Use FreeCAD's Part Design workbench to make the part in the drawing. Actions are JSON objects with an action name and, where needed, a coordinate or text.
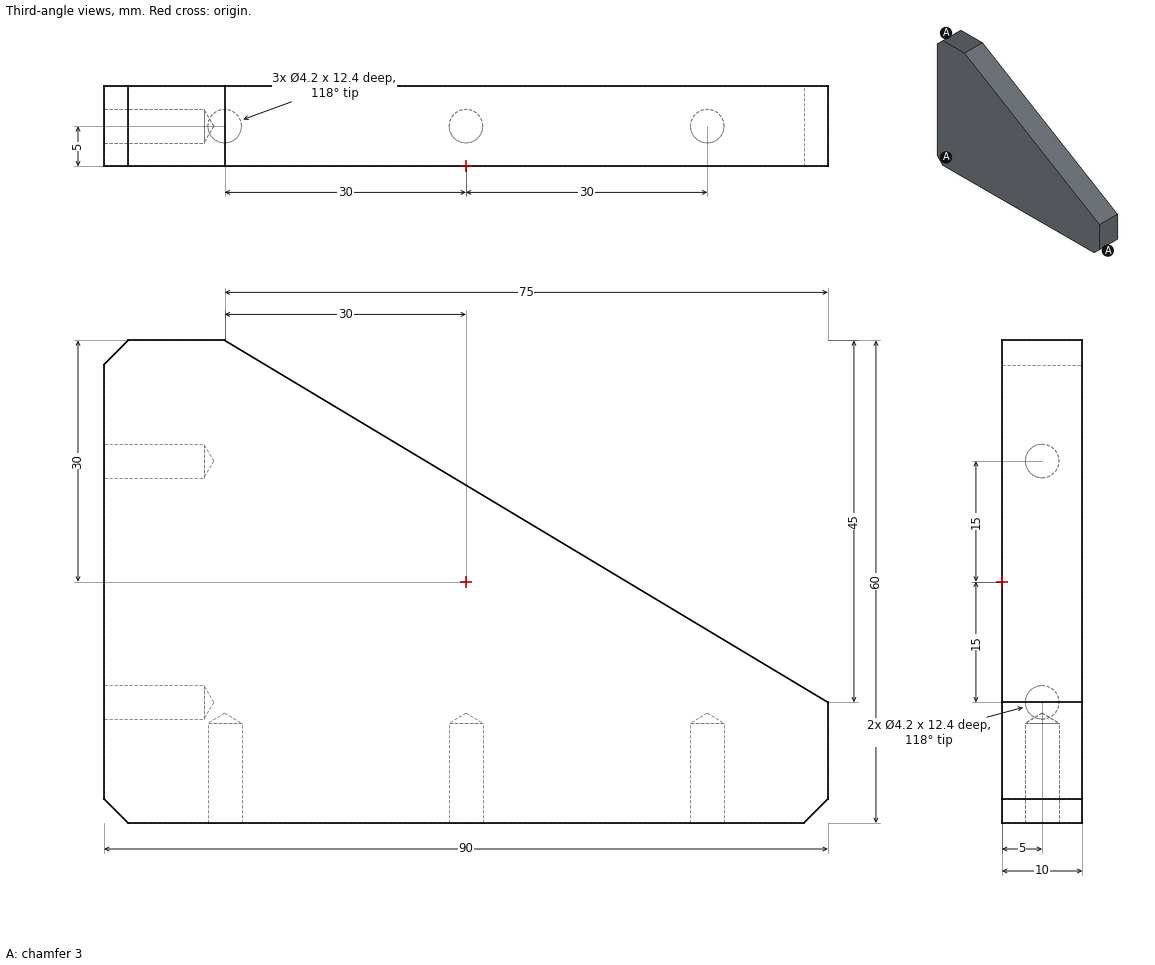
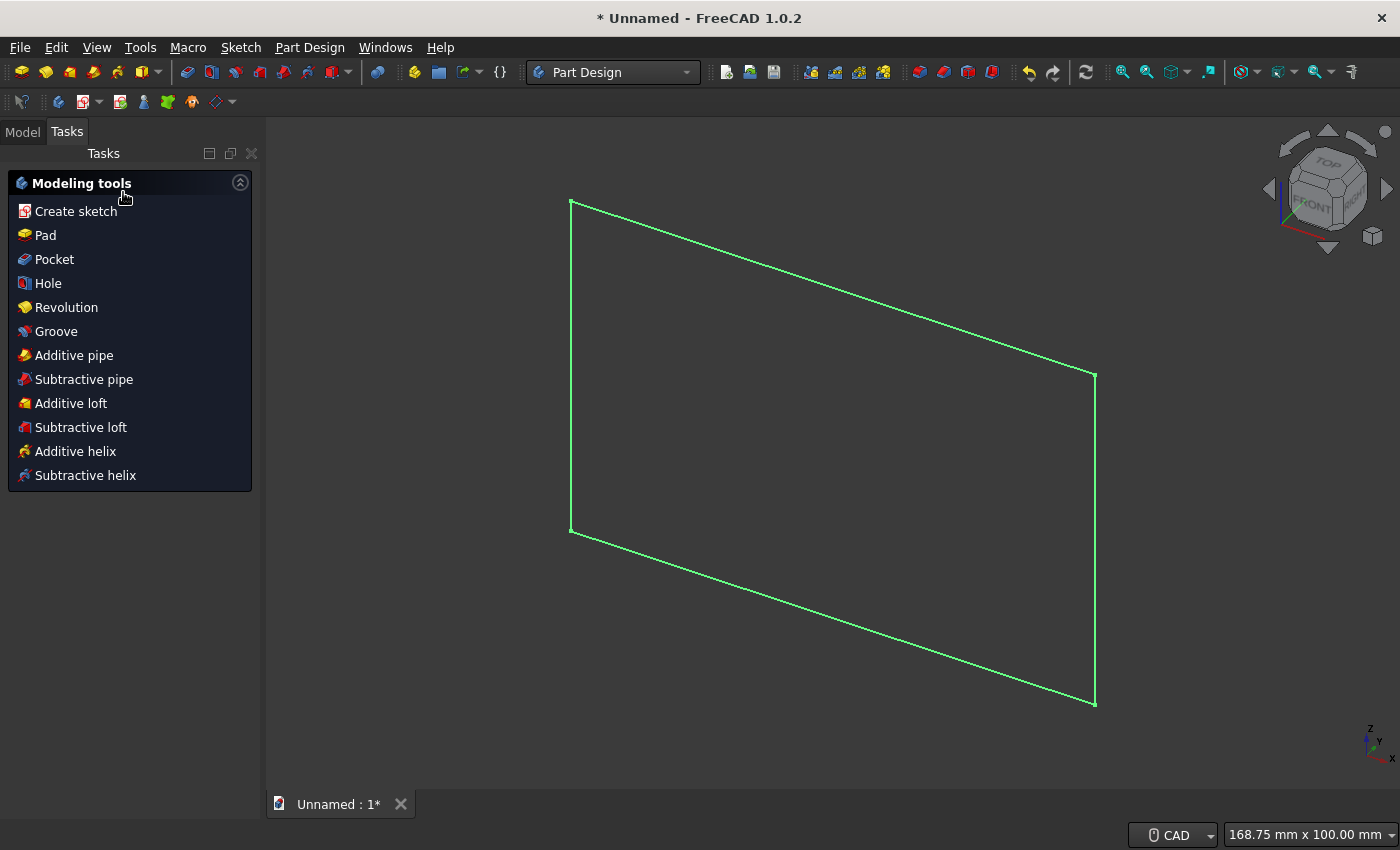
{"action": "left_click", "coordinate": [22, 72]}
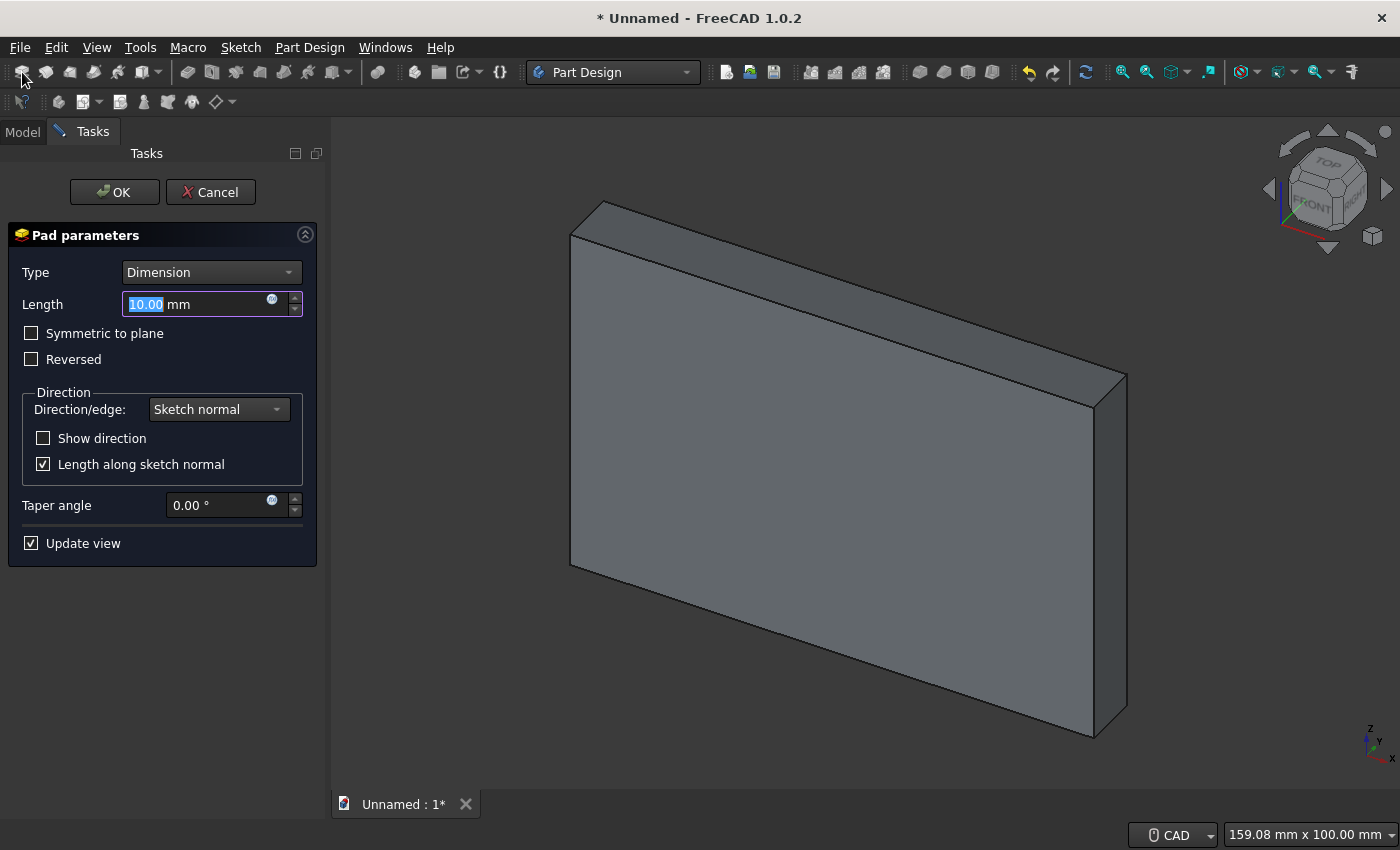
{"action": "type", "text": "10"}
{"action": "key", "text": "Tab"}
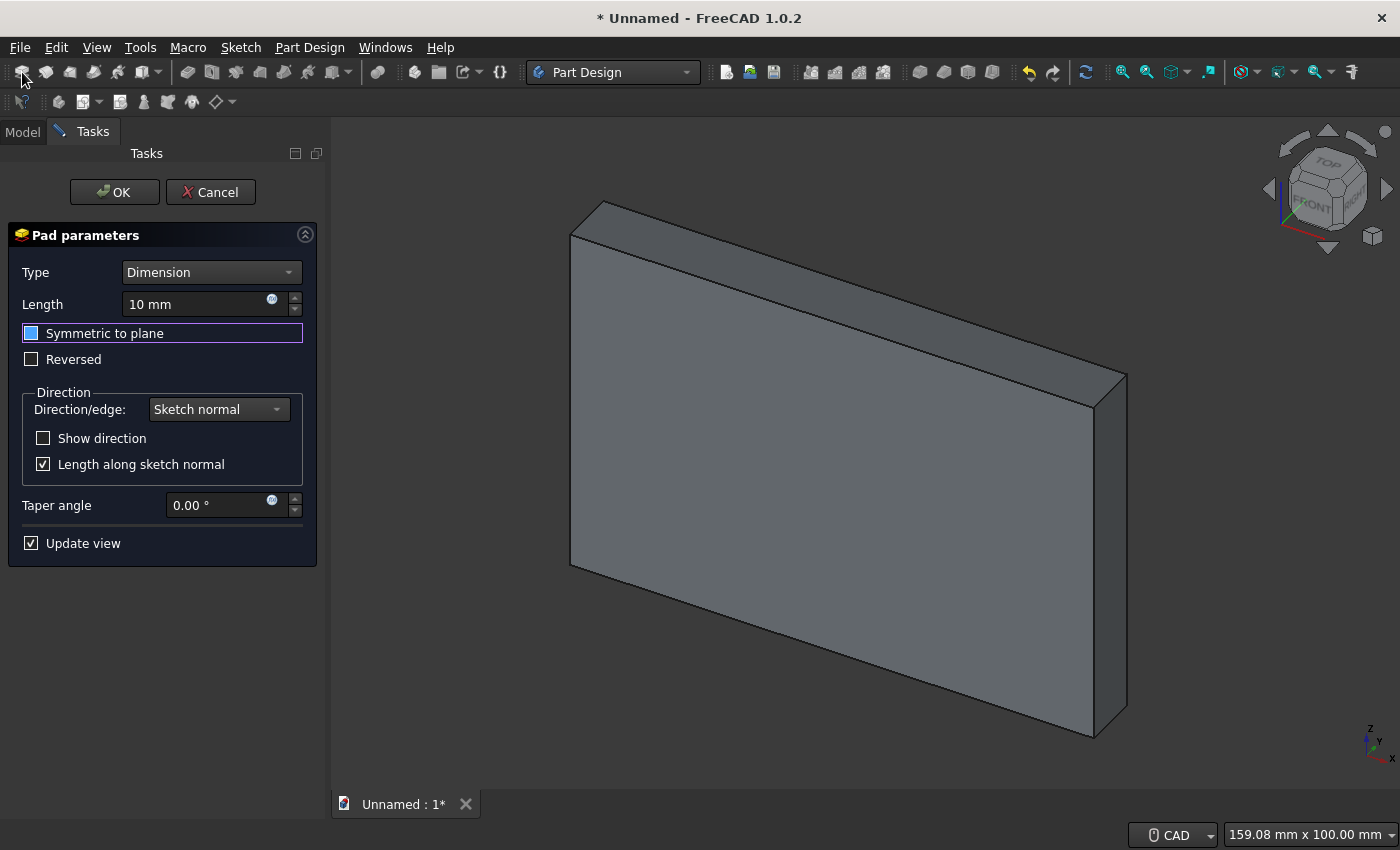
{"action": "left_click", "coordinate": [30, 359]}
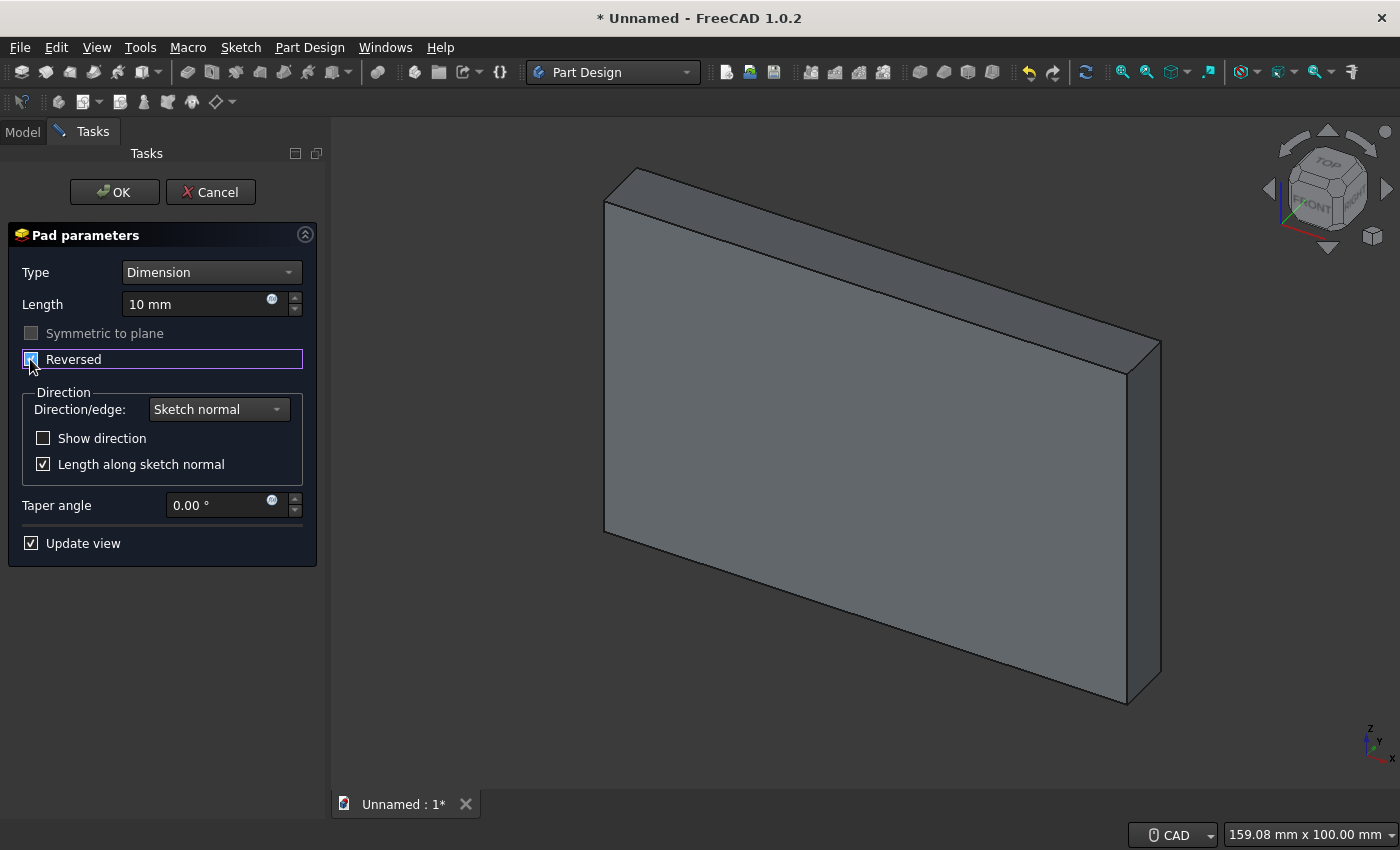
{"action": "left_click", "coordinate": [115, 192]}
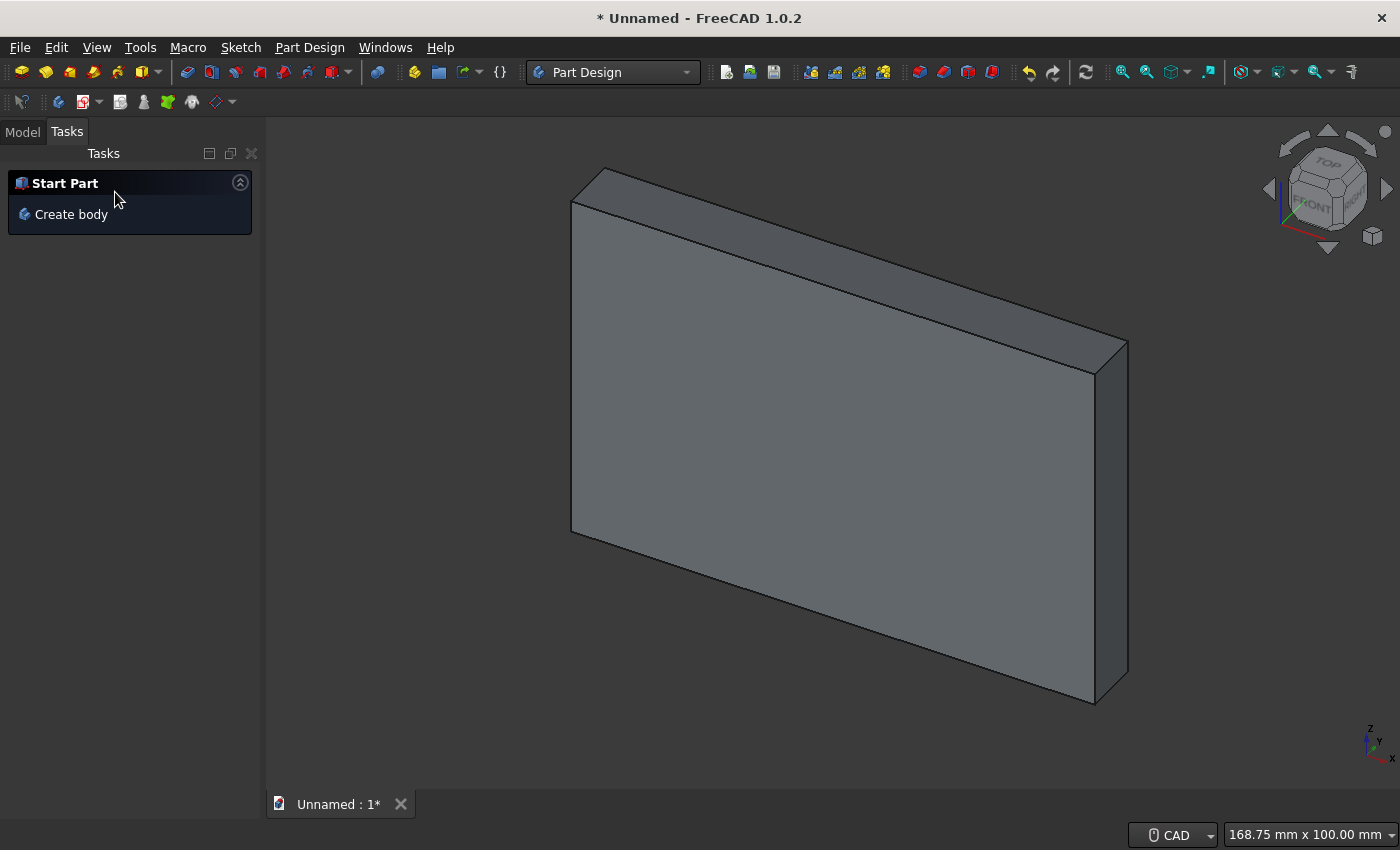
{"action": "key", "text": "4"}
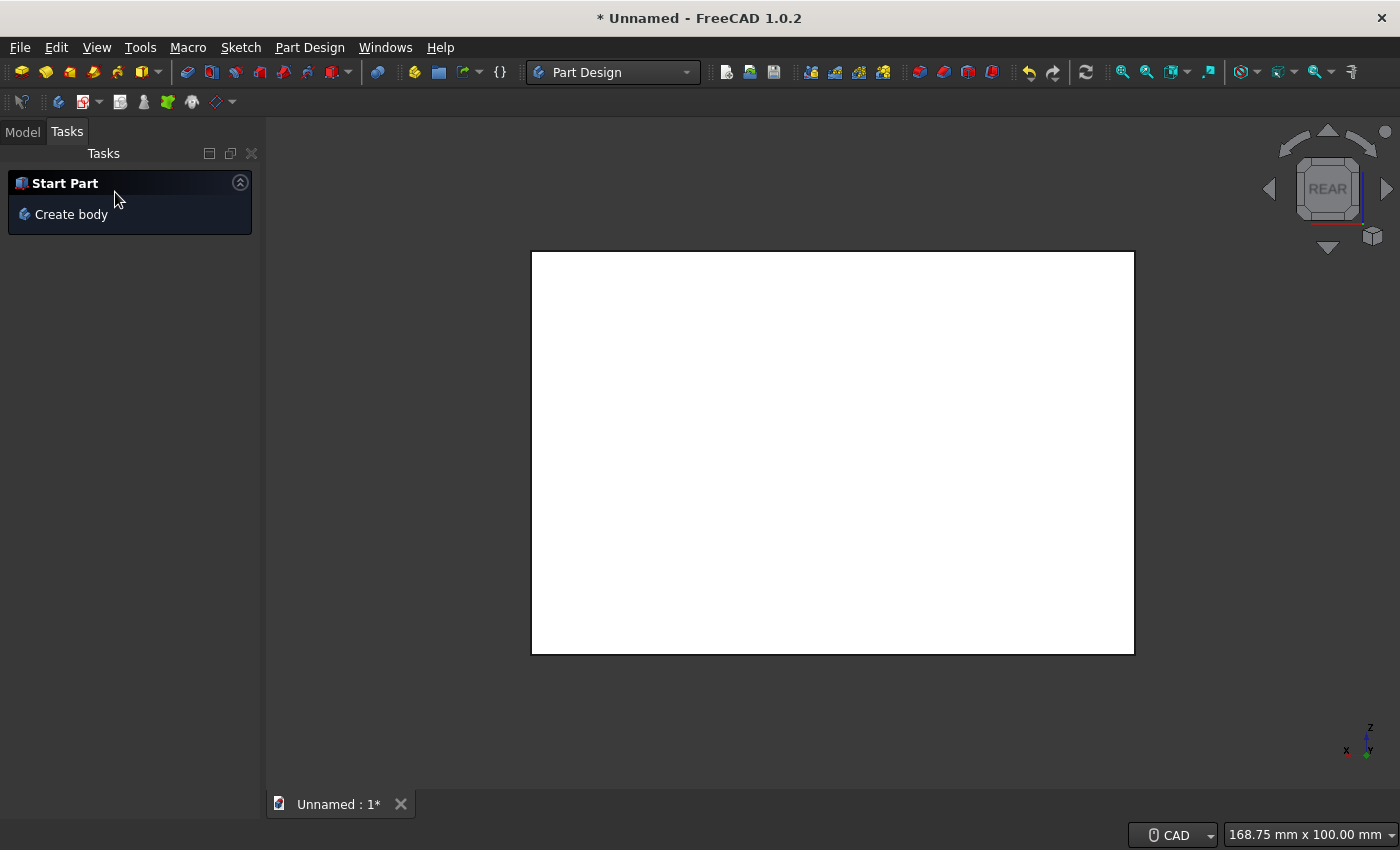
{"action": "left_click", "coordinate": [747, 452]}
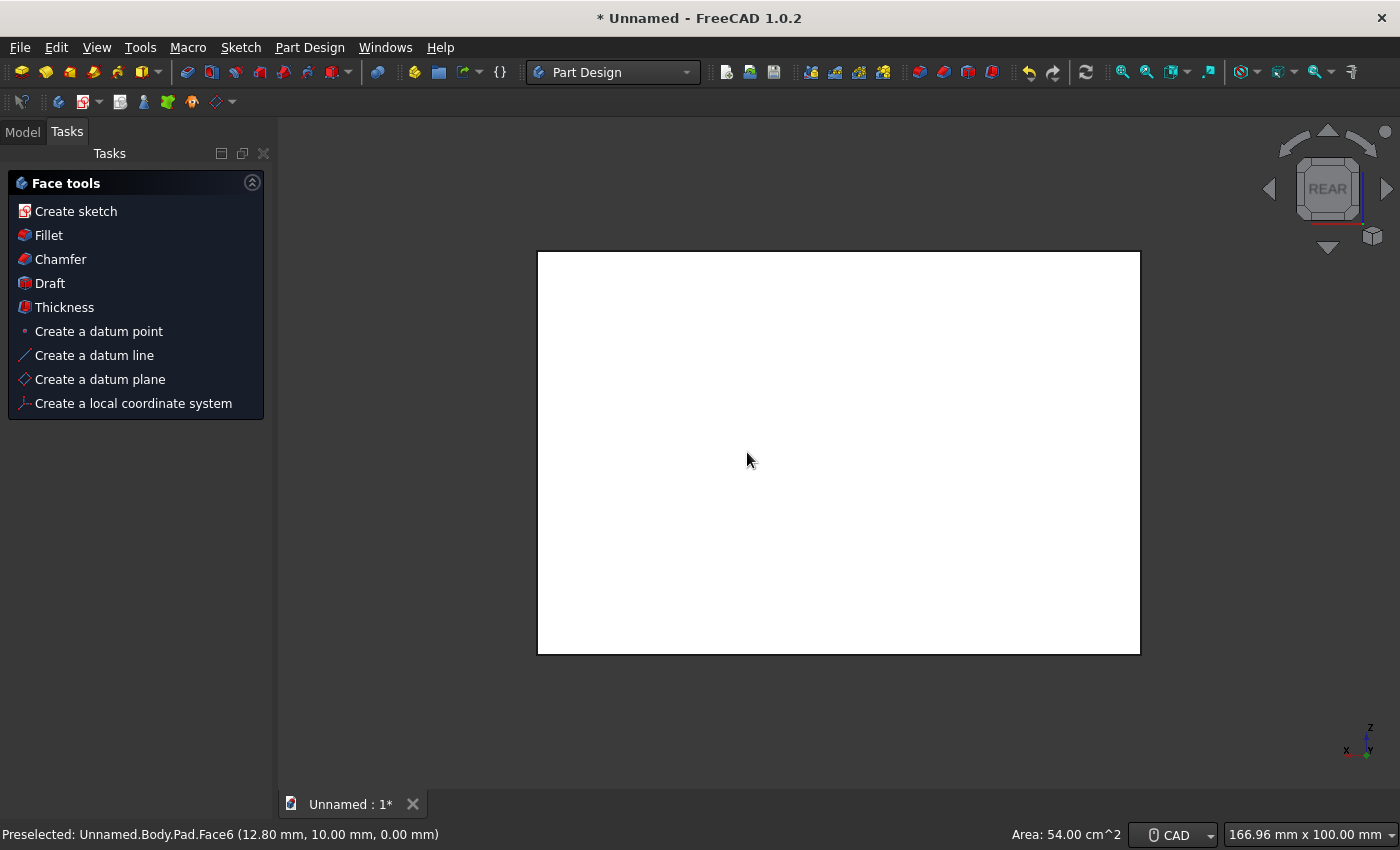
{"action": "left_click", "coordinate": [84, 102]}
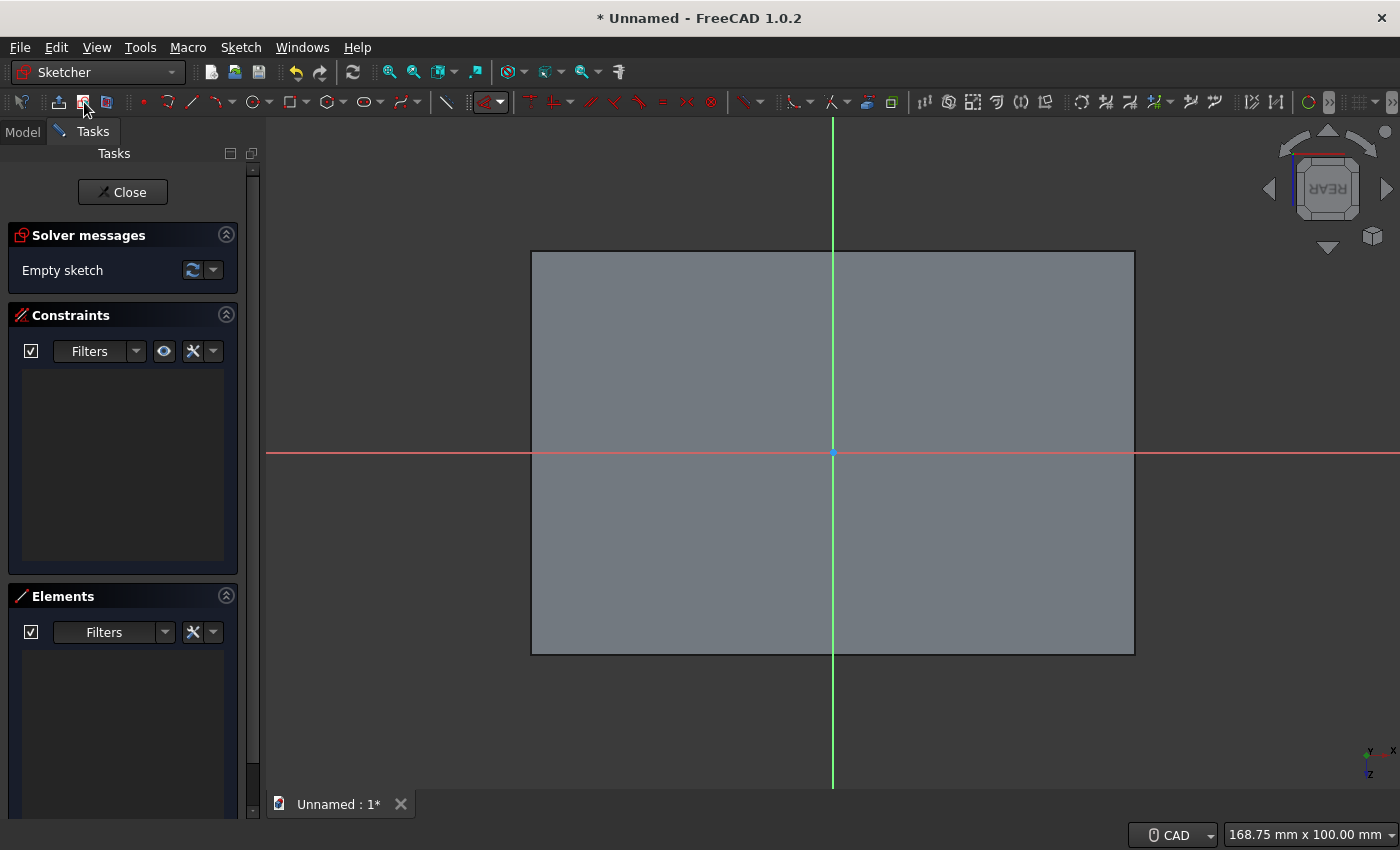
{"action": "key", "text": "g m"}